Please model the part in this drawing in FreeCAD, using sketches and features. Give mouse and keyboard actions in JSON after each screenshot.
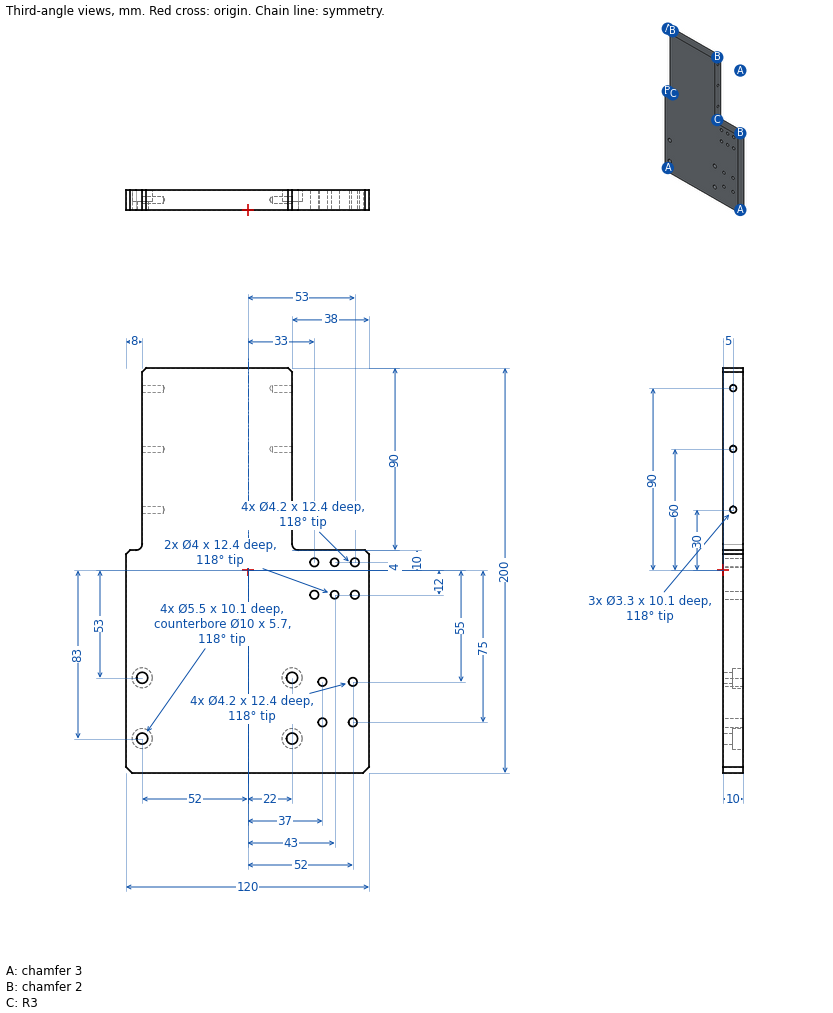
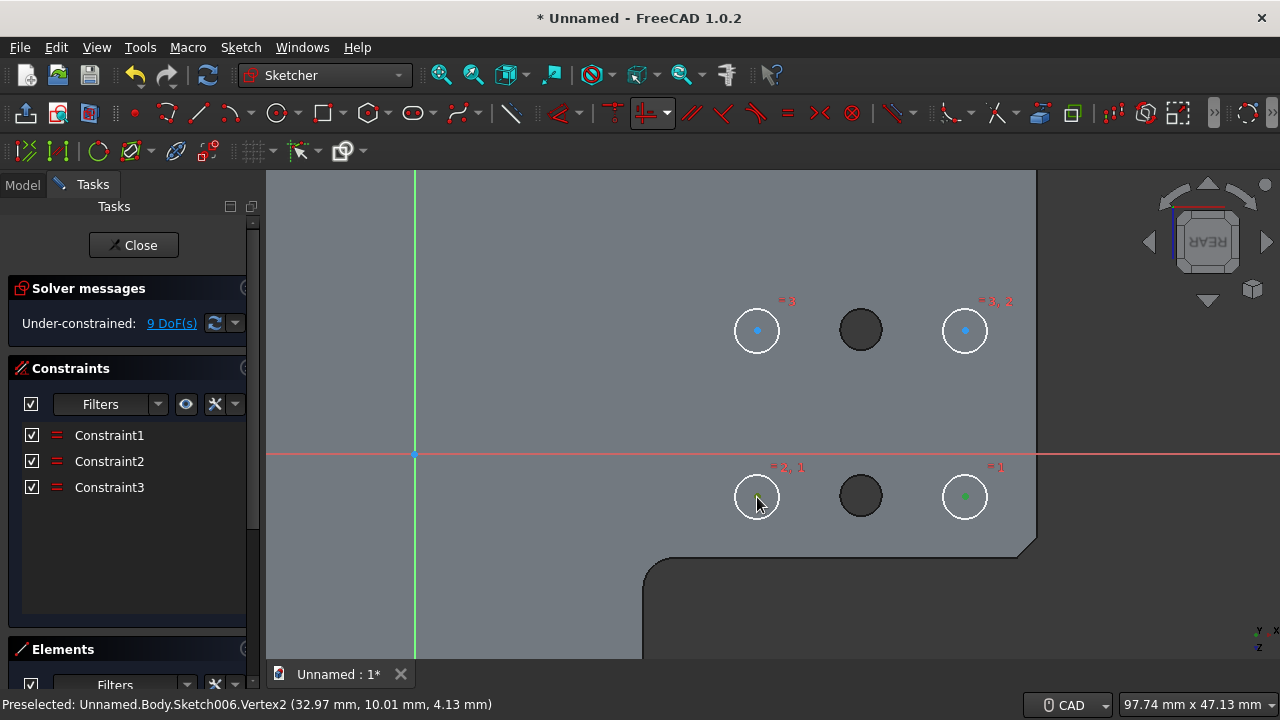
{"action": "key", "text": "h"}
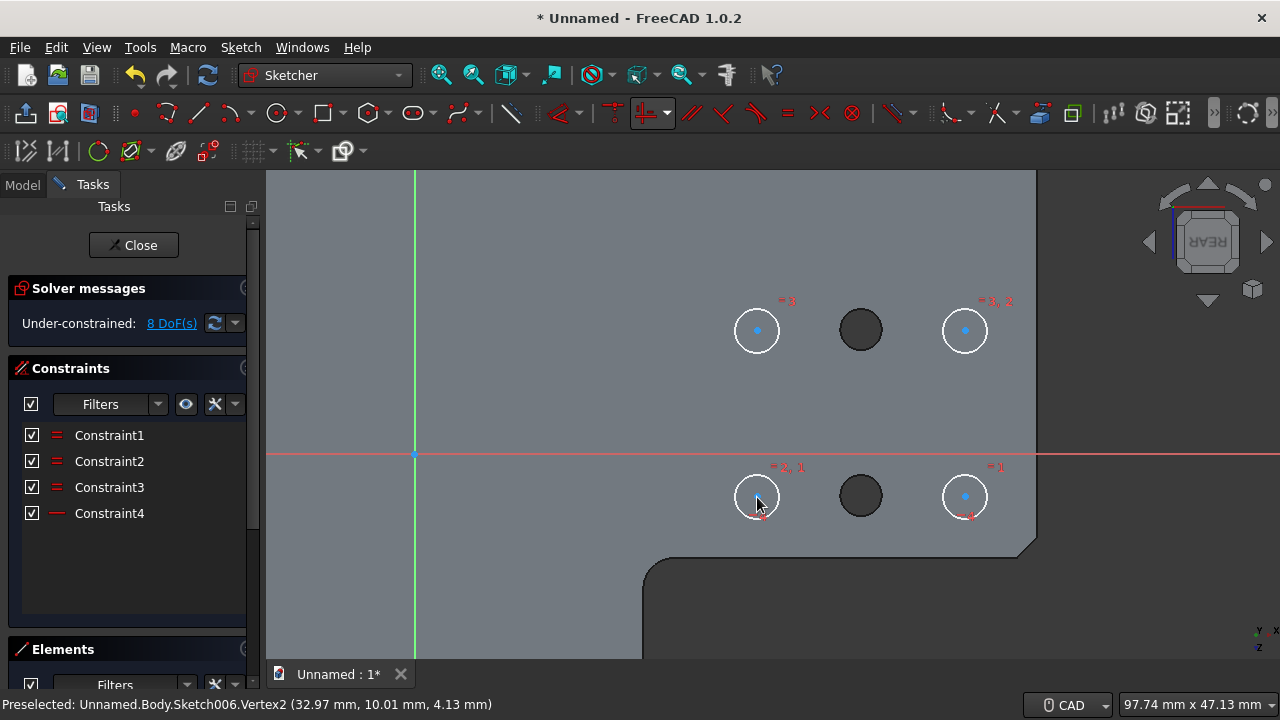
{"action": "left_click", "coordinate": [965, 497]}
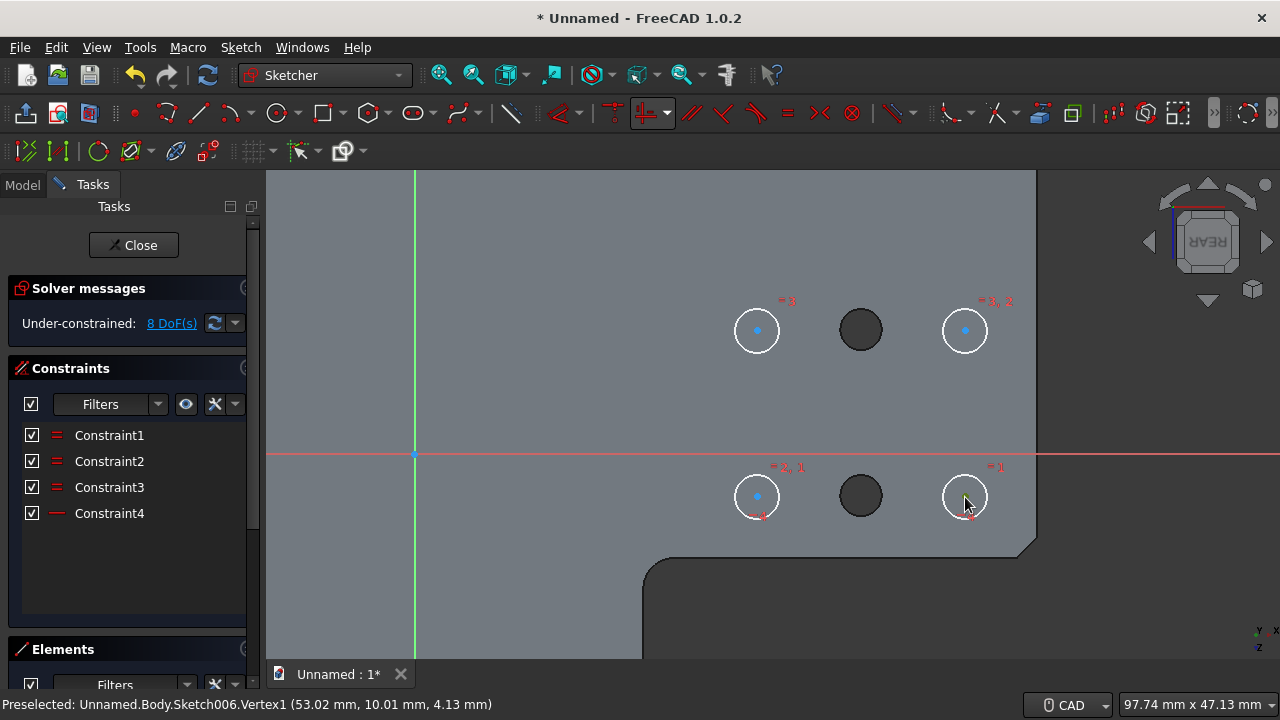
{"action": "left_click", "coordinate": [965, 331]}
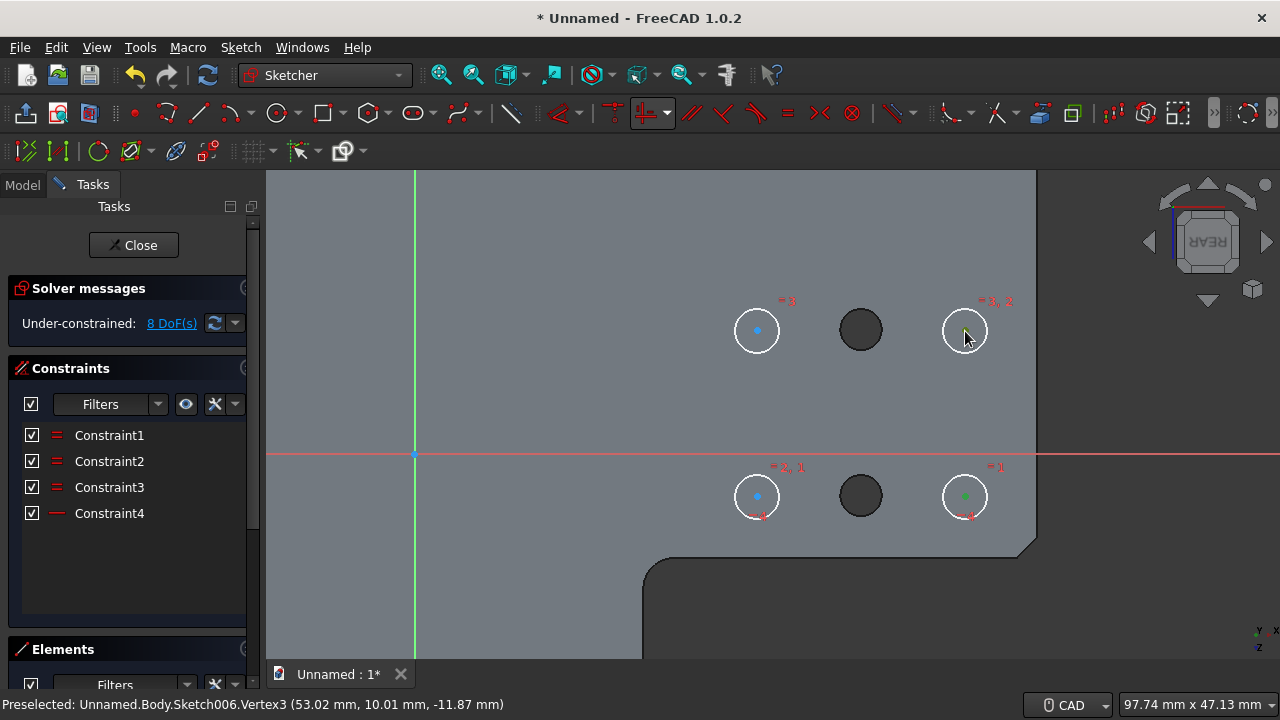
{"action": "left_click", "coordinate": [670, 114]}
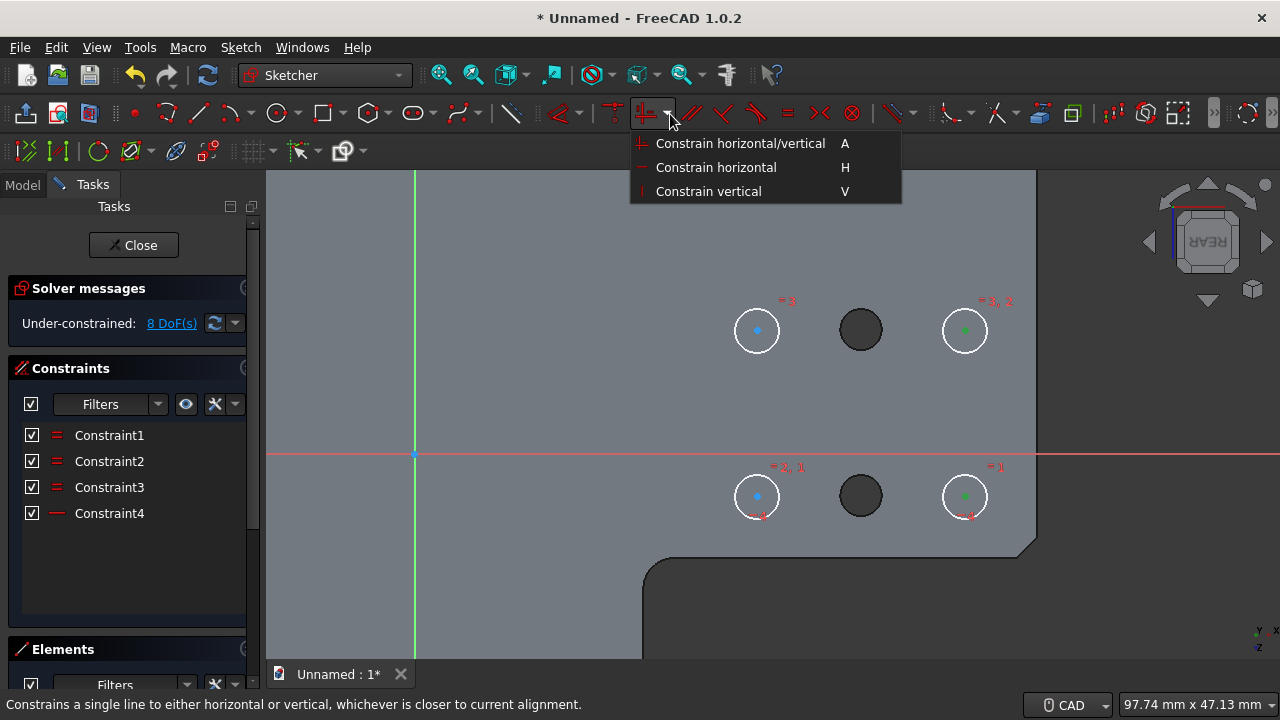
{"action": "left_click", "coordinate": [766, 191]}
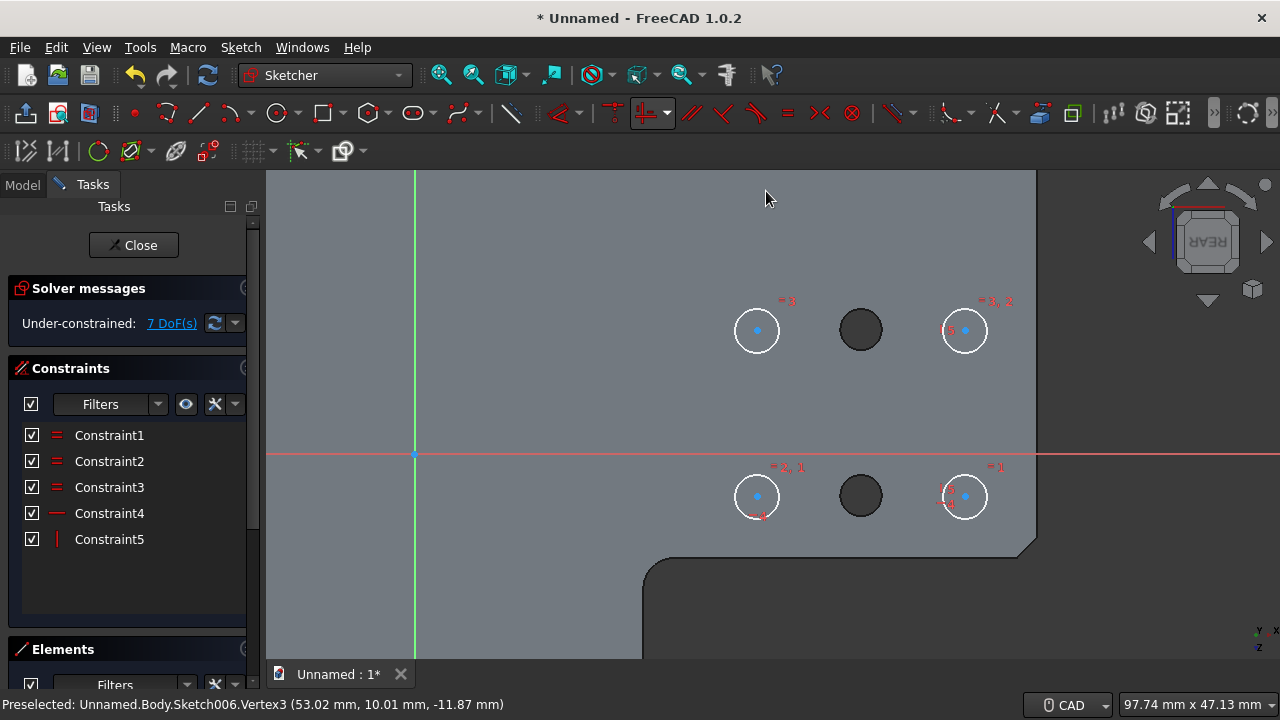
{"action": "left_click", "coordinate": [757, 497]}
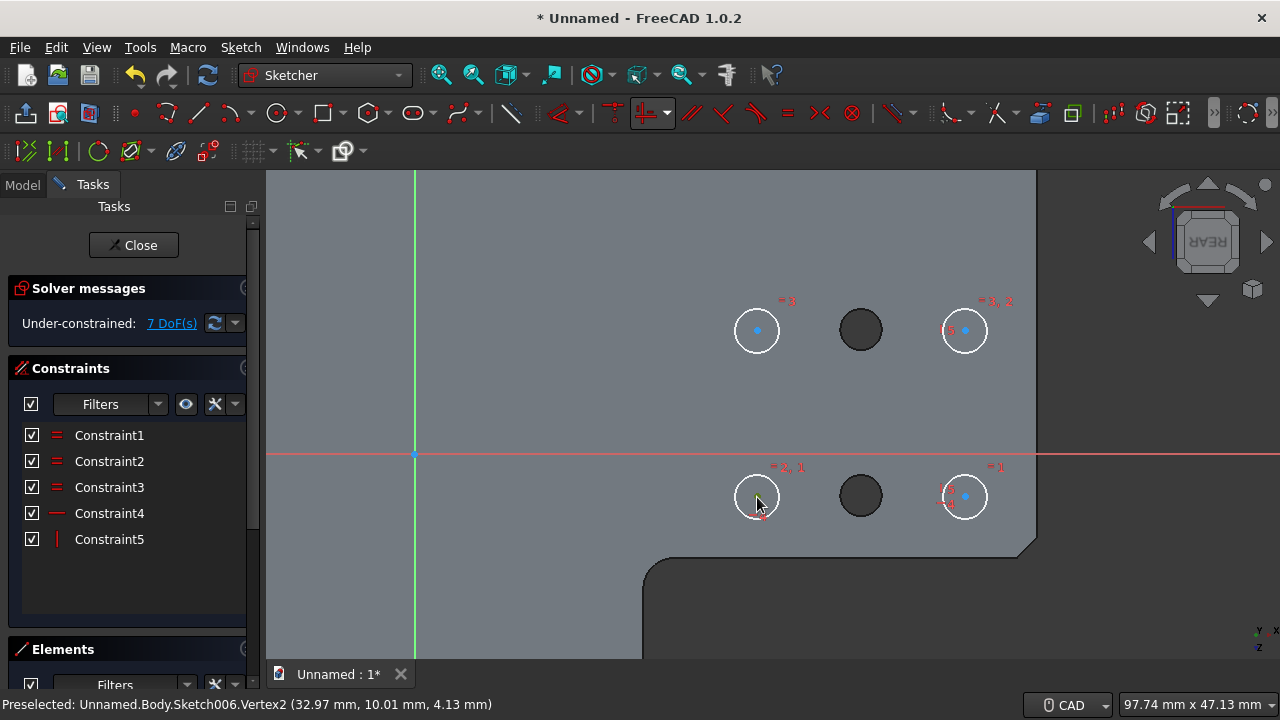
{"action": "left_click", "coordinate": [757, 331]}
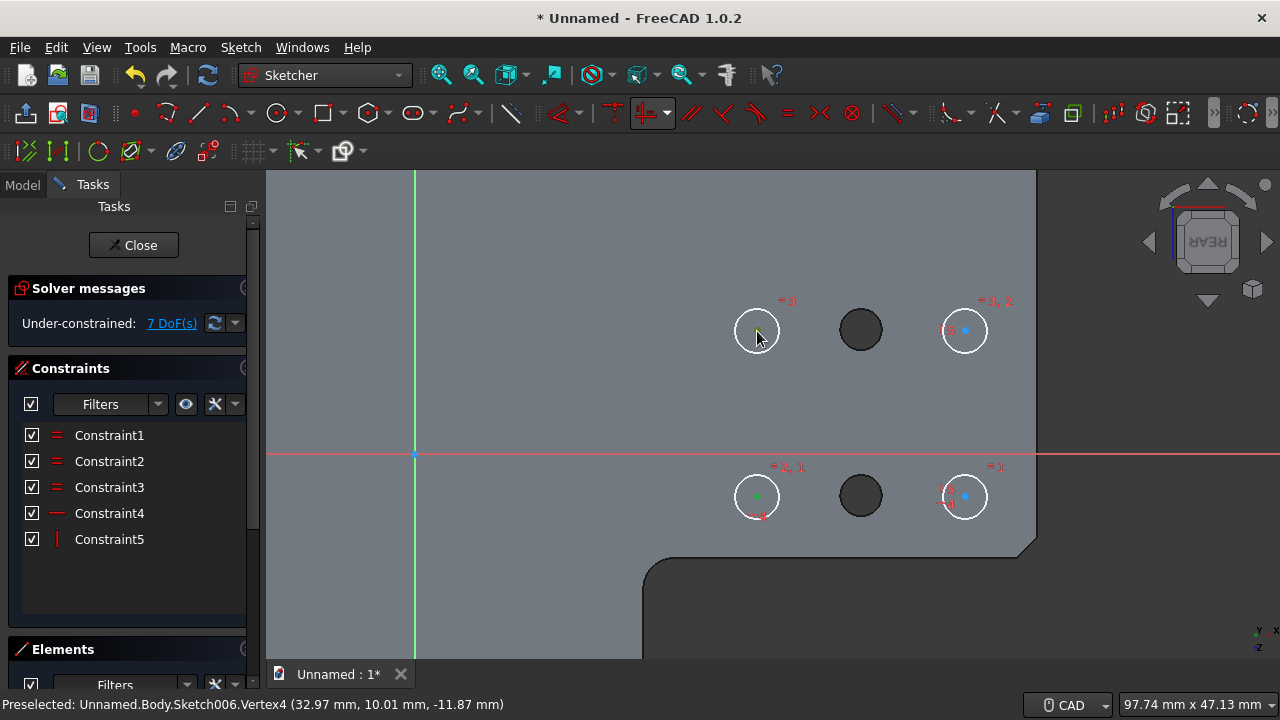
{"action": "left_click", "coordinate": [670, 114]}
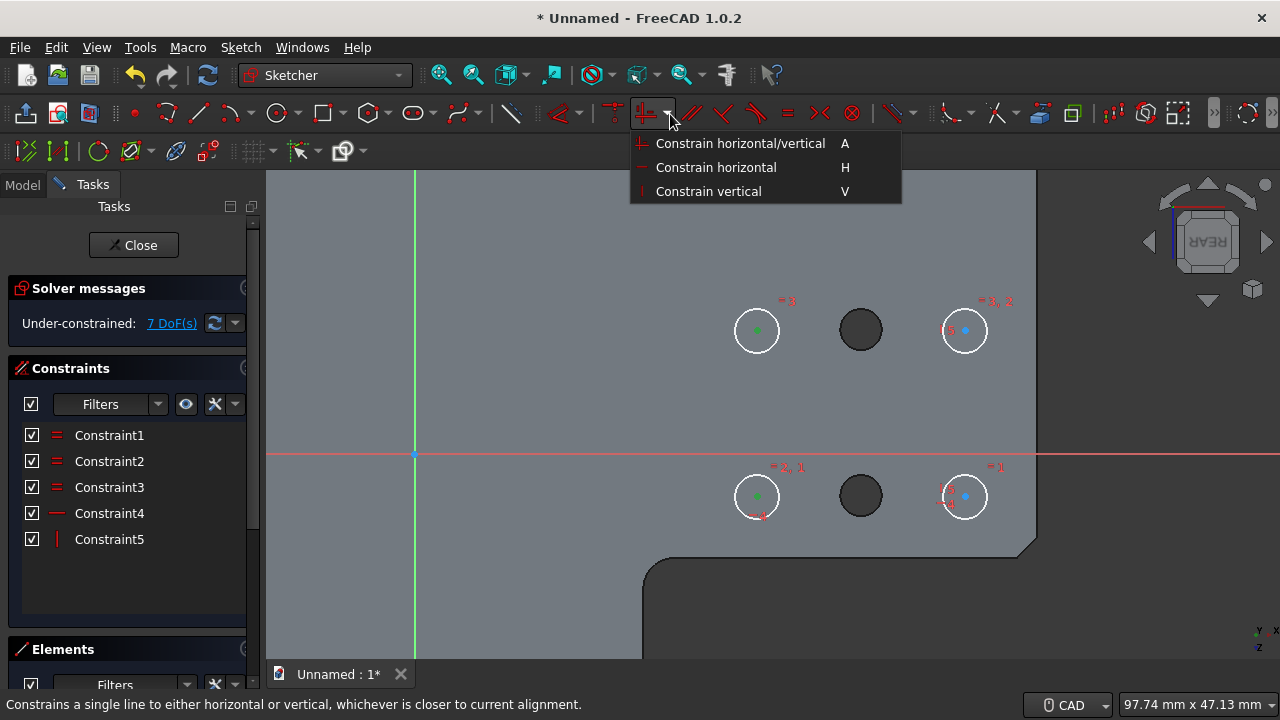
{"action": "left_click", "coordinate": [766, 191]}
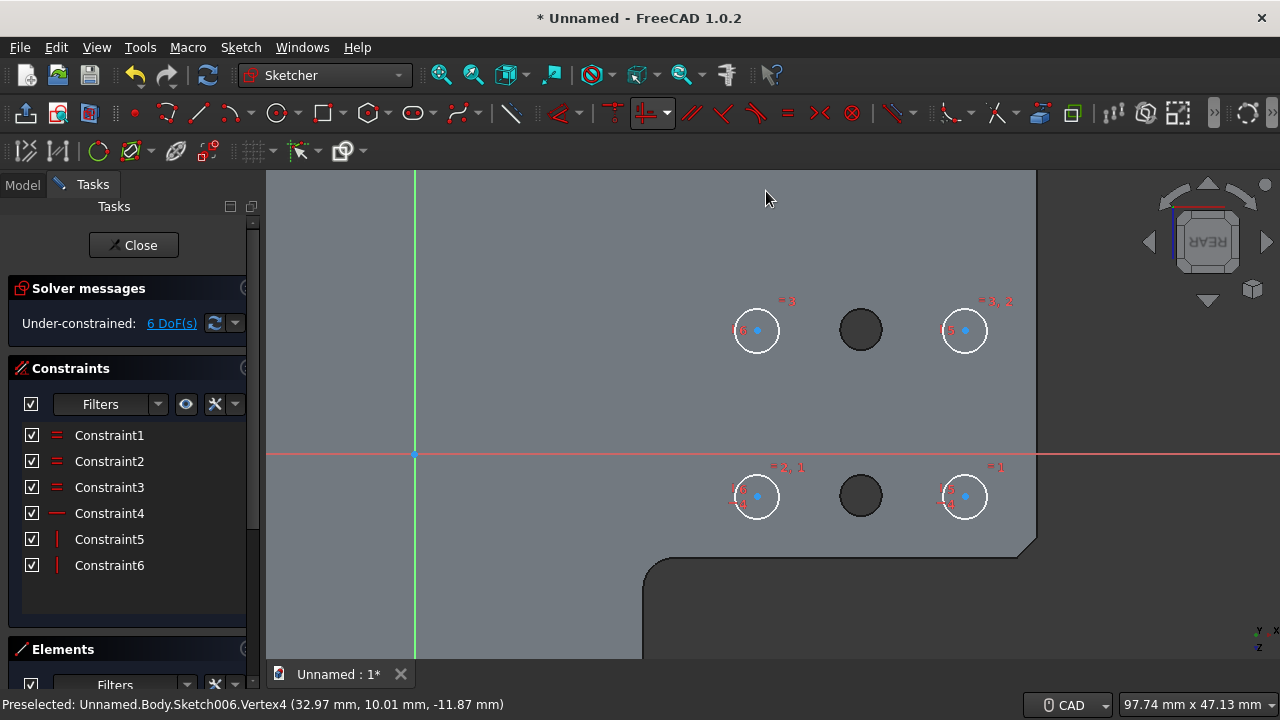
{"action": "left_click", "coordinate": [965, 331]}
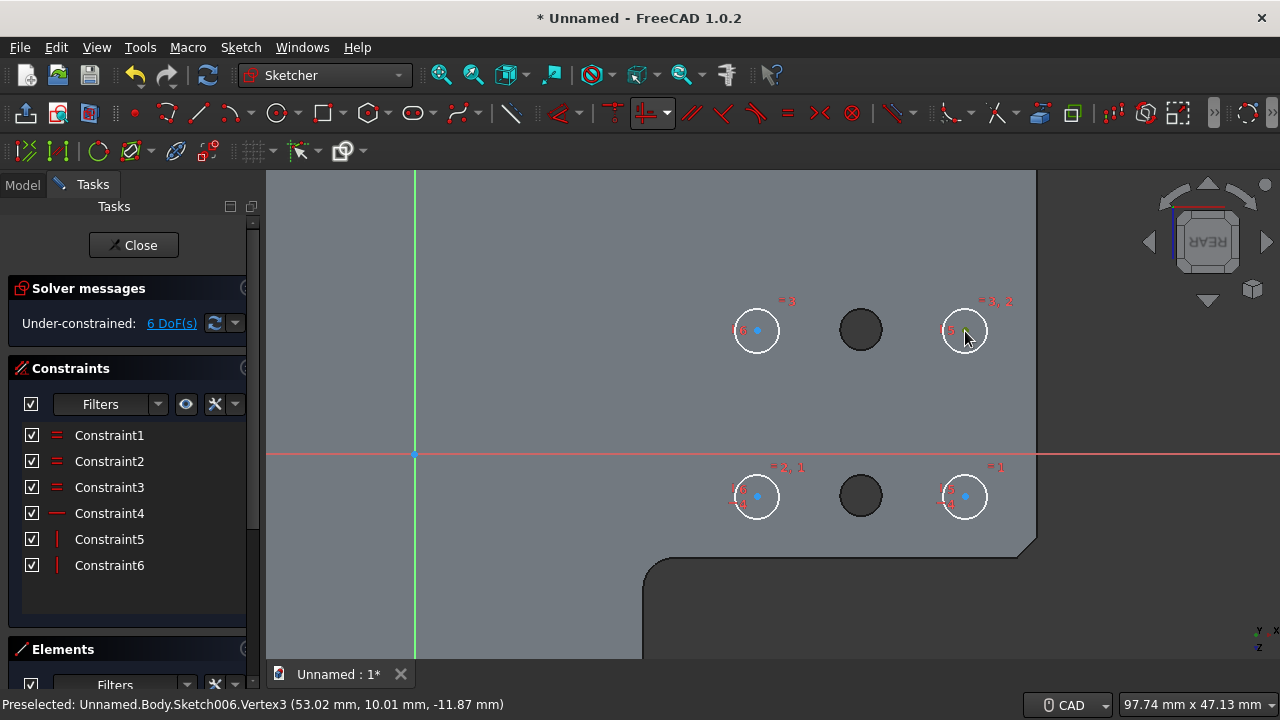
{"action": "left_click", "coordinate": [757, 331]}